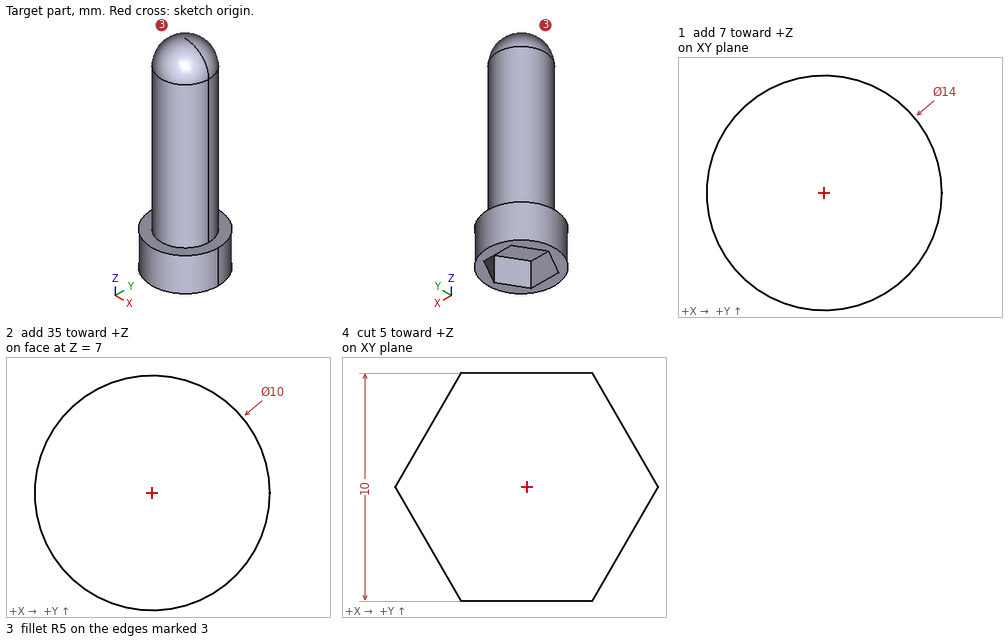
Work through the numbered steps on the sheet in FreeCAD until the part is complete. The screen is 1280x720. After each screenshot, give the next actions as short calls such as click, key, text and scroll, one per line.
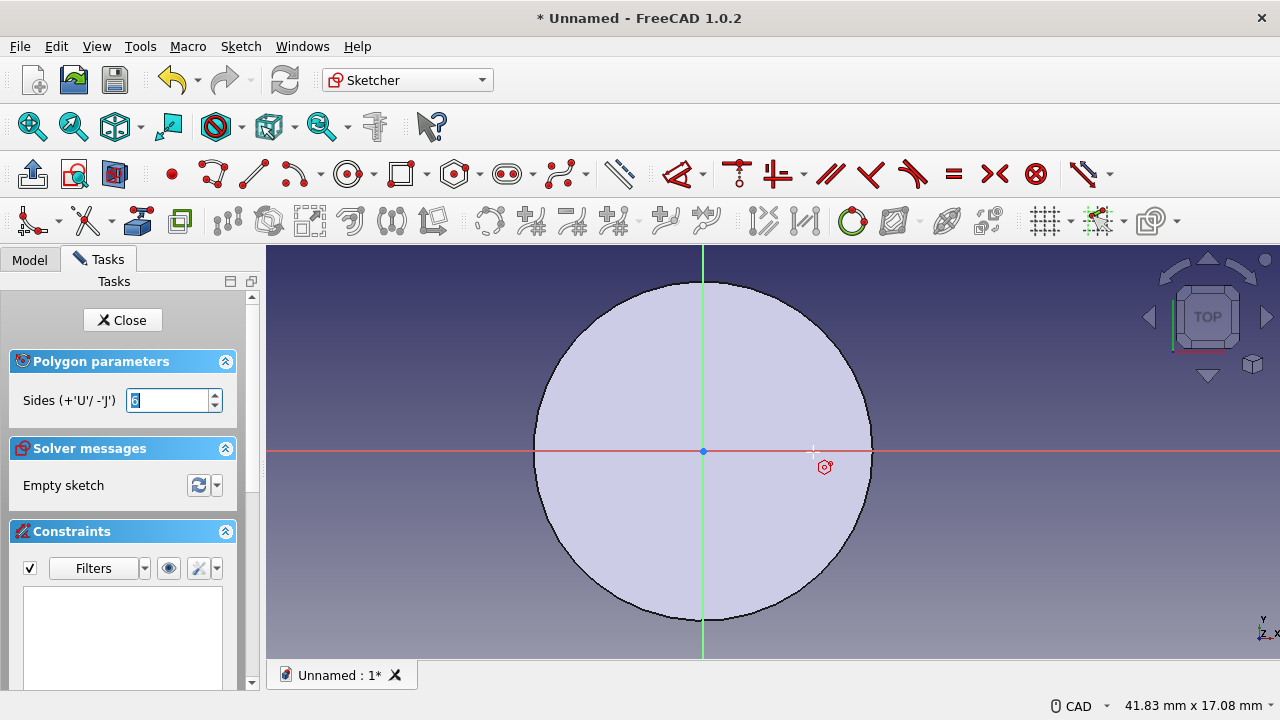
click(703, 451)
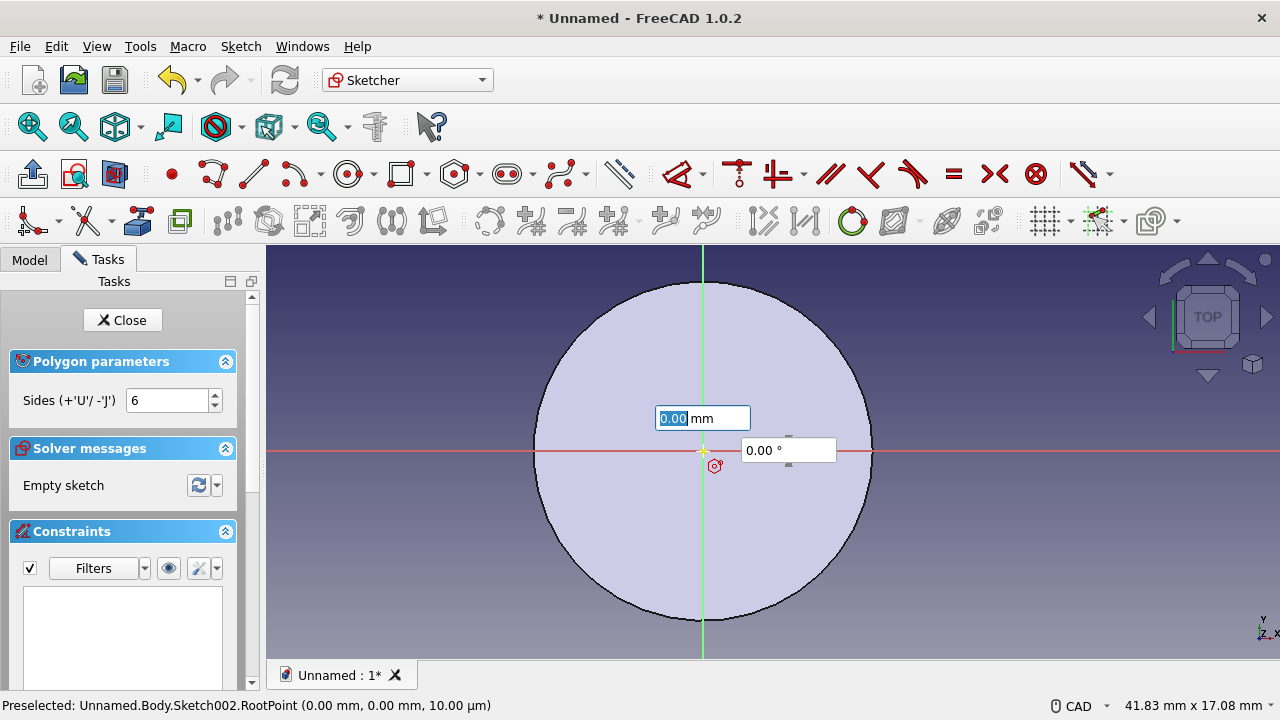
click(563, 451)
right_click(563, 451)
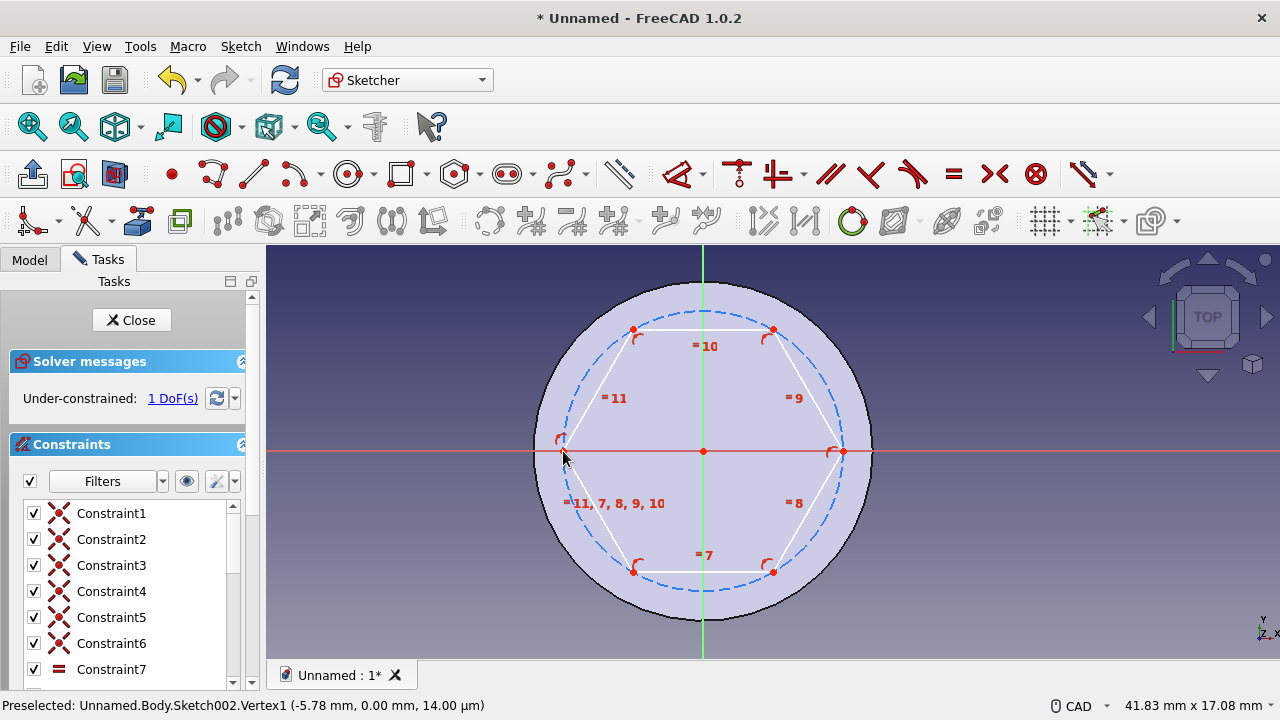
key(d)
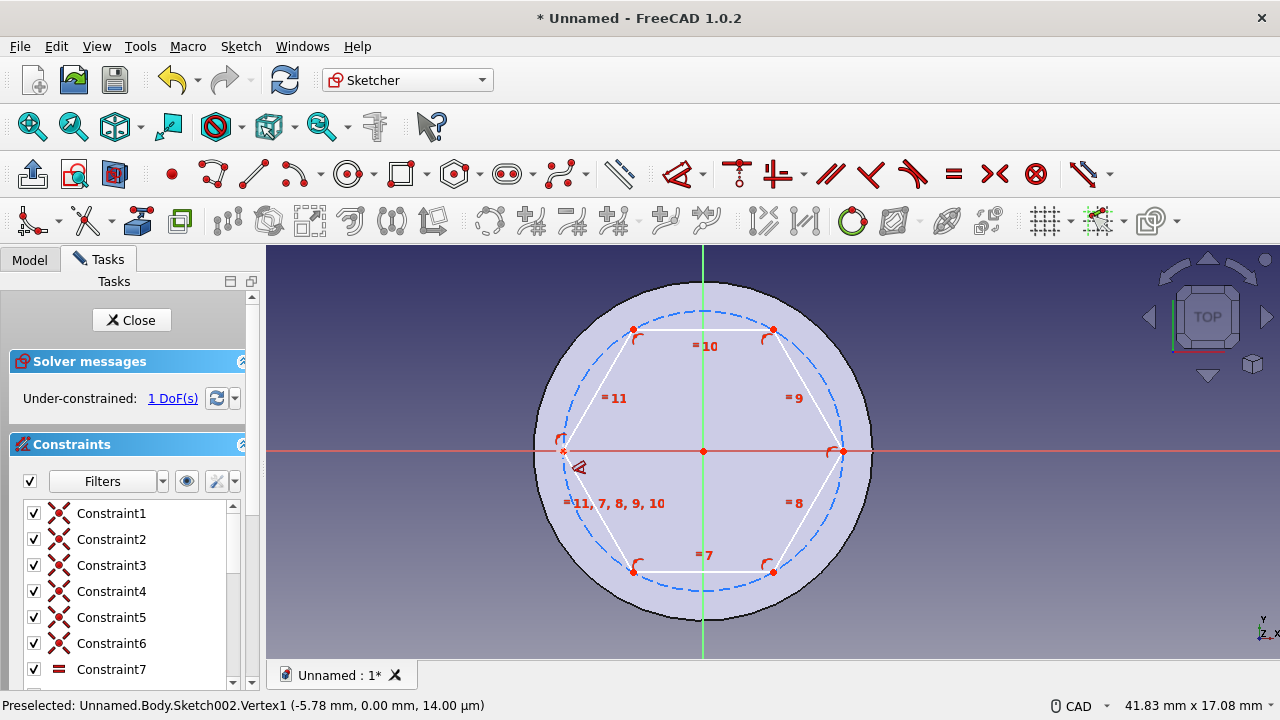
click(633, 572)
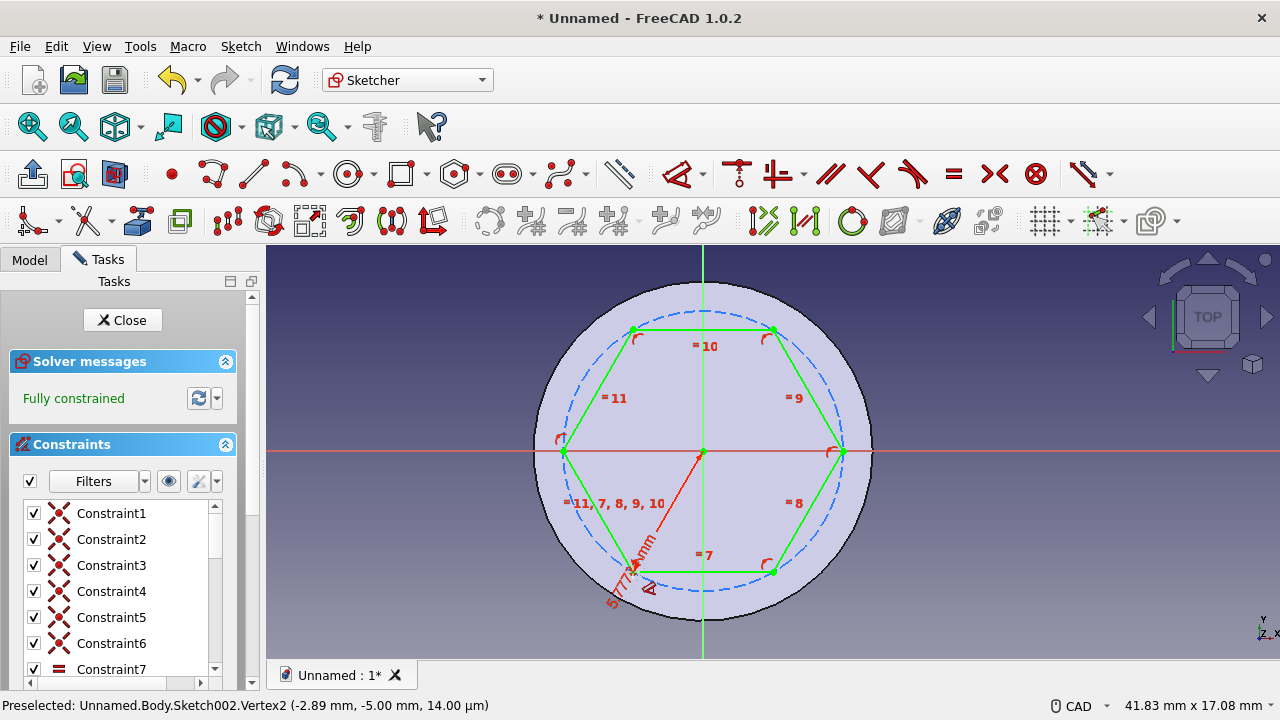
click(773, 330)
click(831, 366)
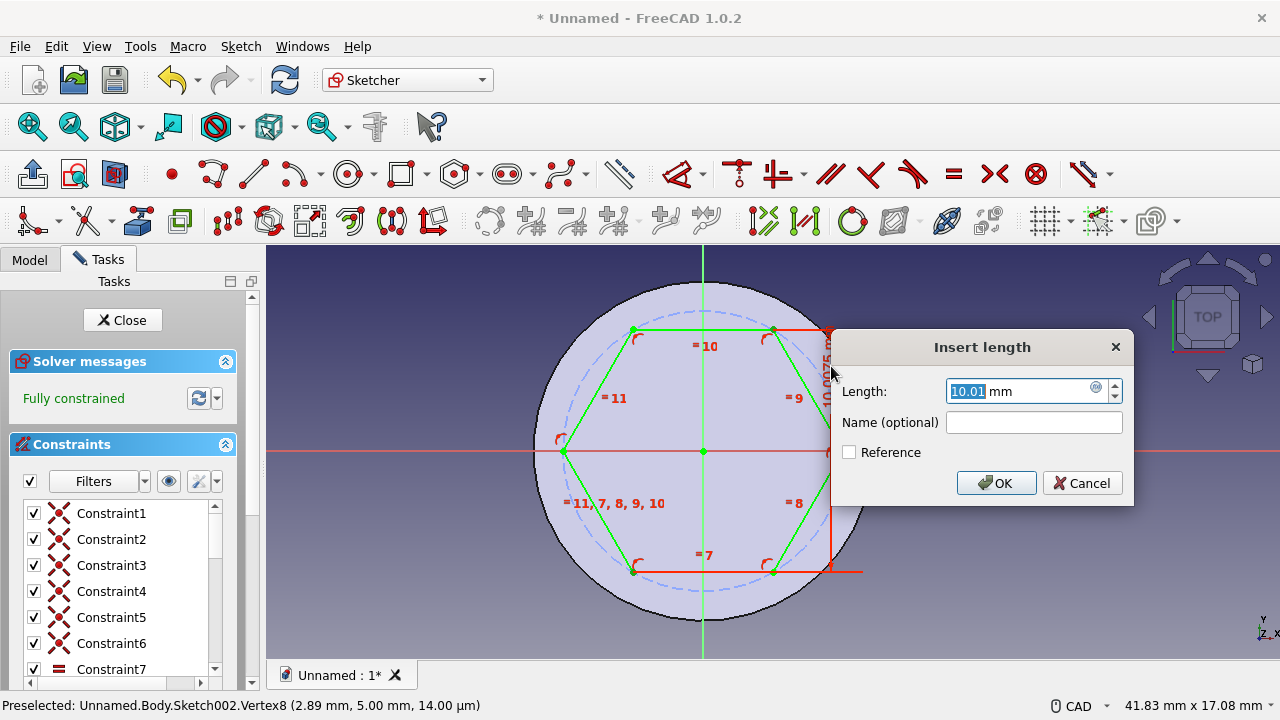
text(10)
key(Return)
key(Escape)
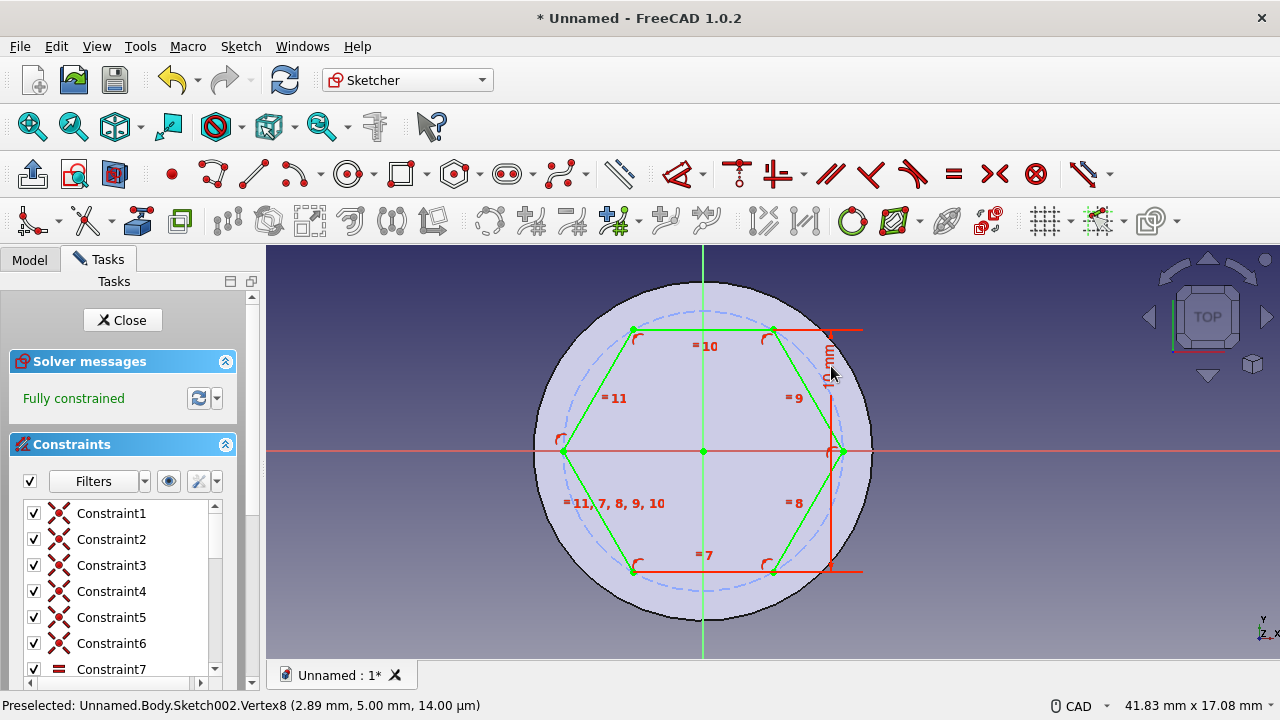
click(123, 320)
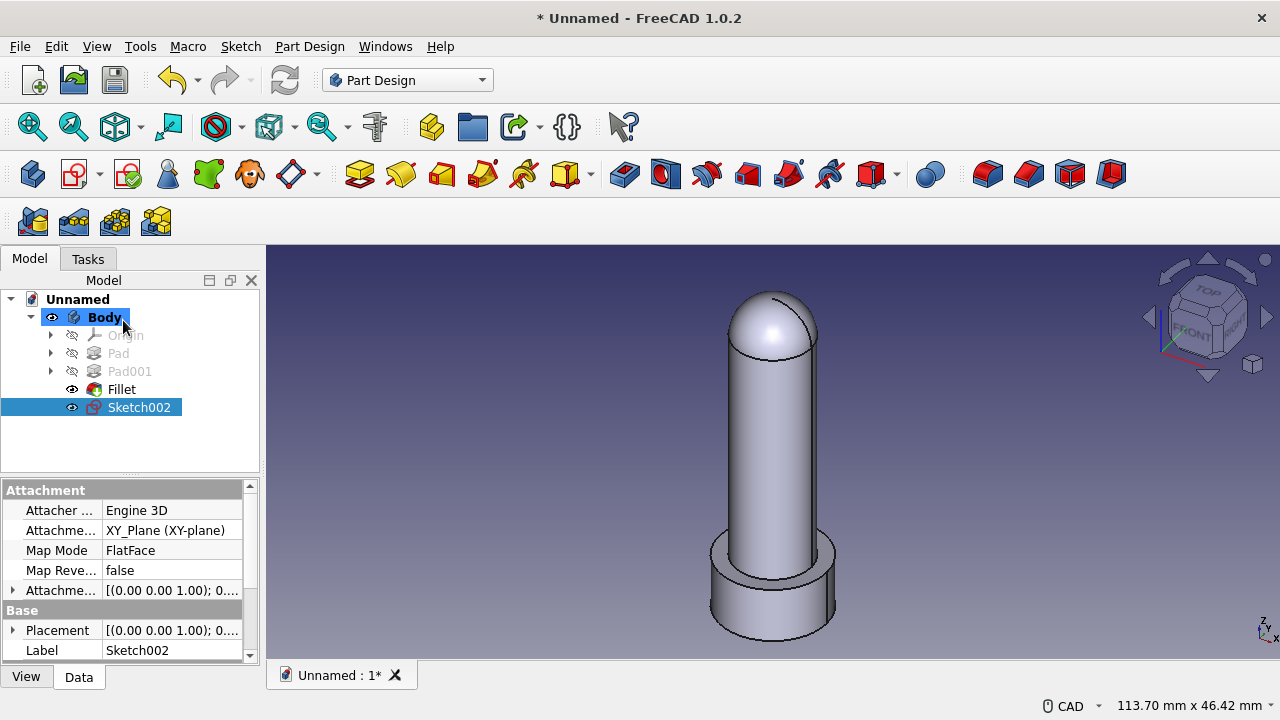
click(625, 174)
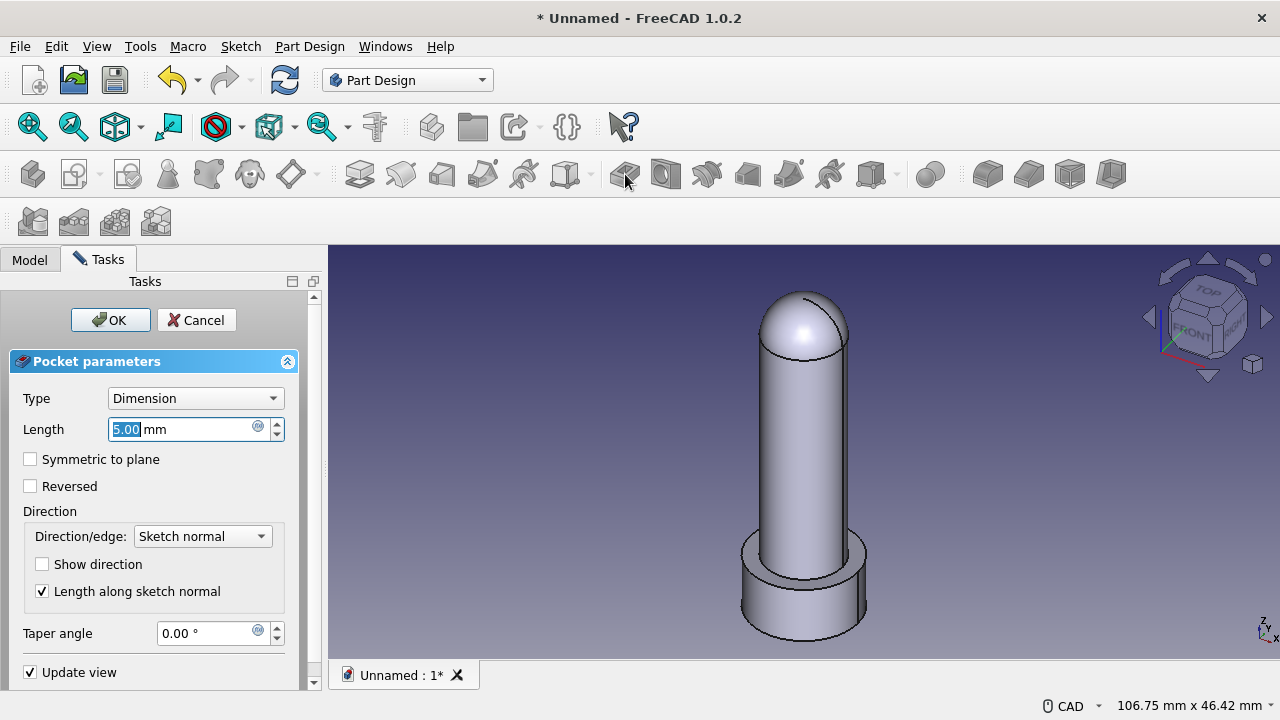
text(5)
key(Tab)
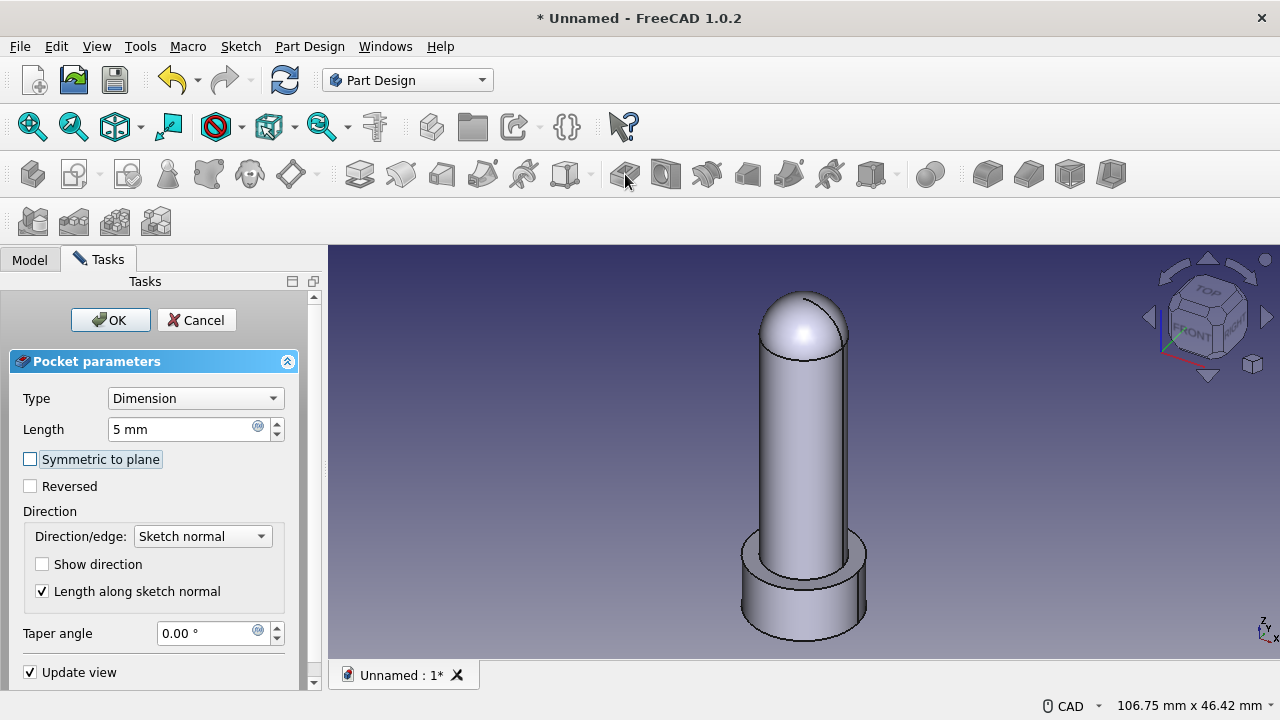
click(31, 486)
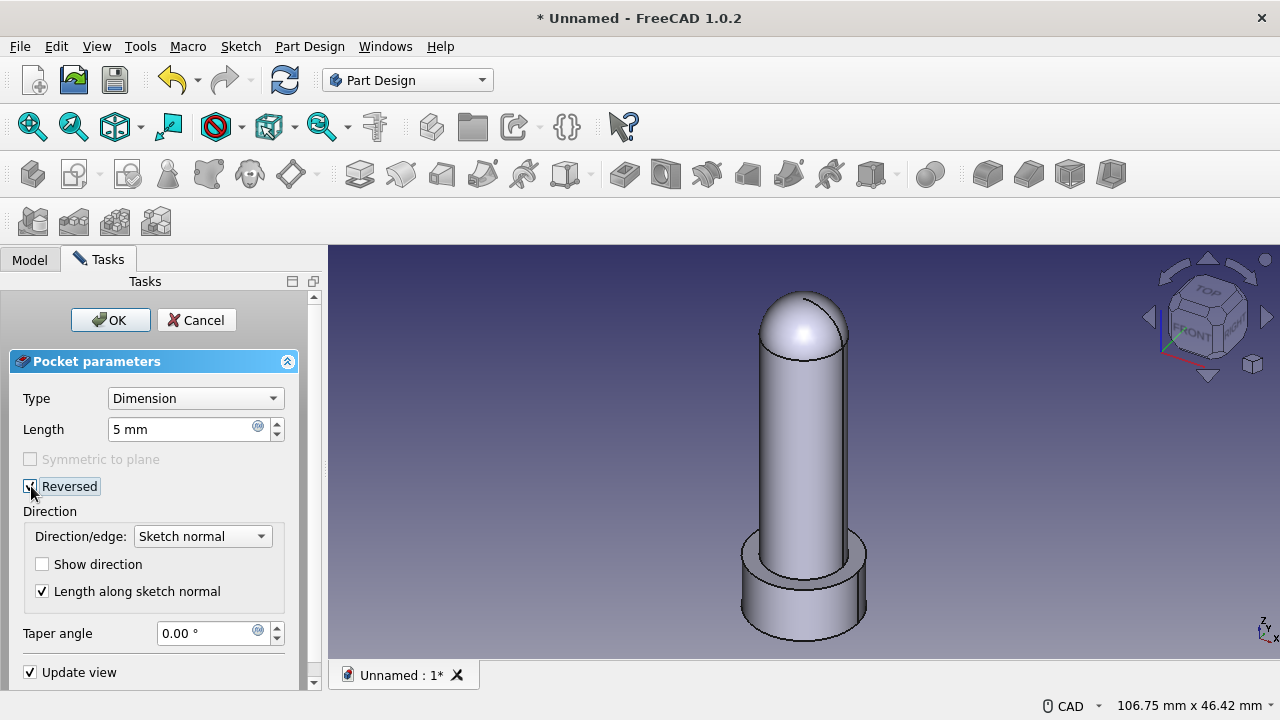
click(111, 320)